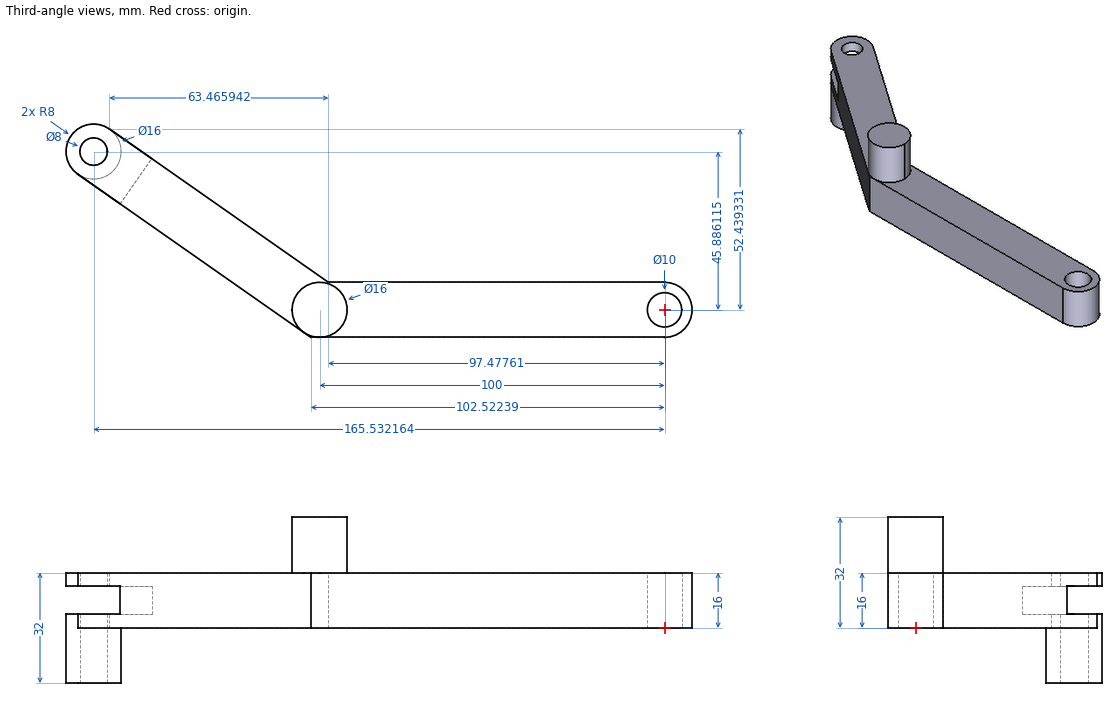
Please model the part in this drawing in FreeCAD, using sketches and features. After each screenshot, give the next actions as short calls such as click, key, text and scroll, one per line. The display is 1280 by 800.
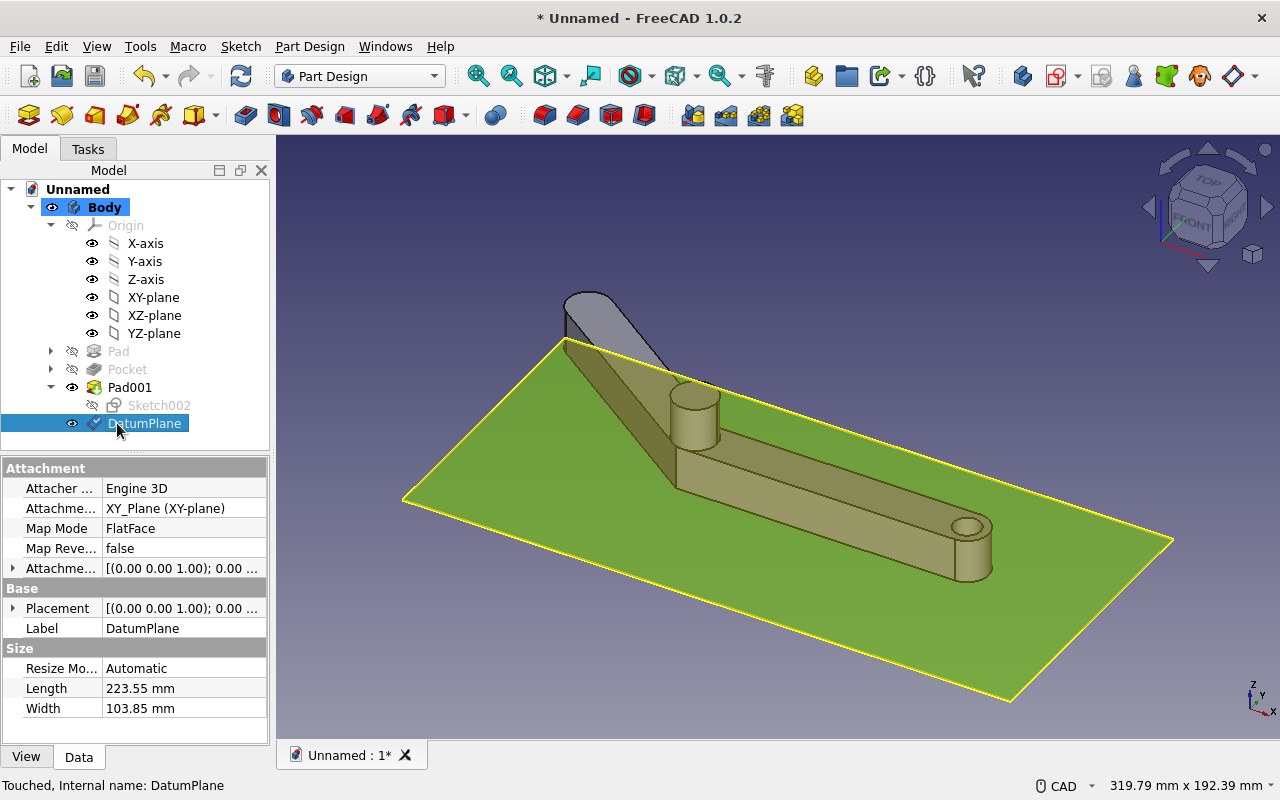
click(1056, 76)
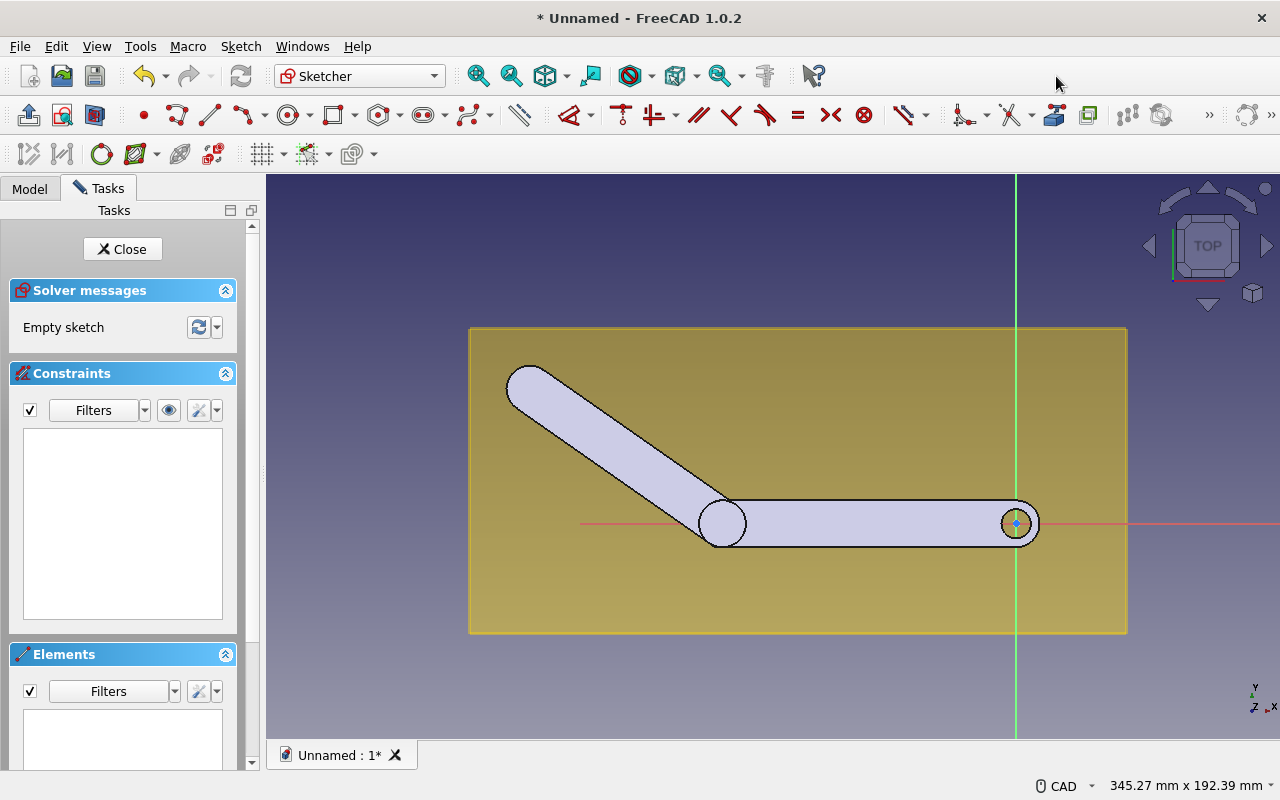
click(95, 116)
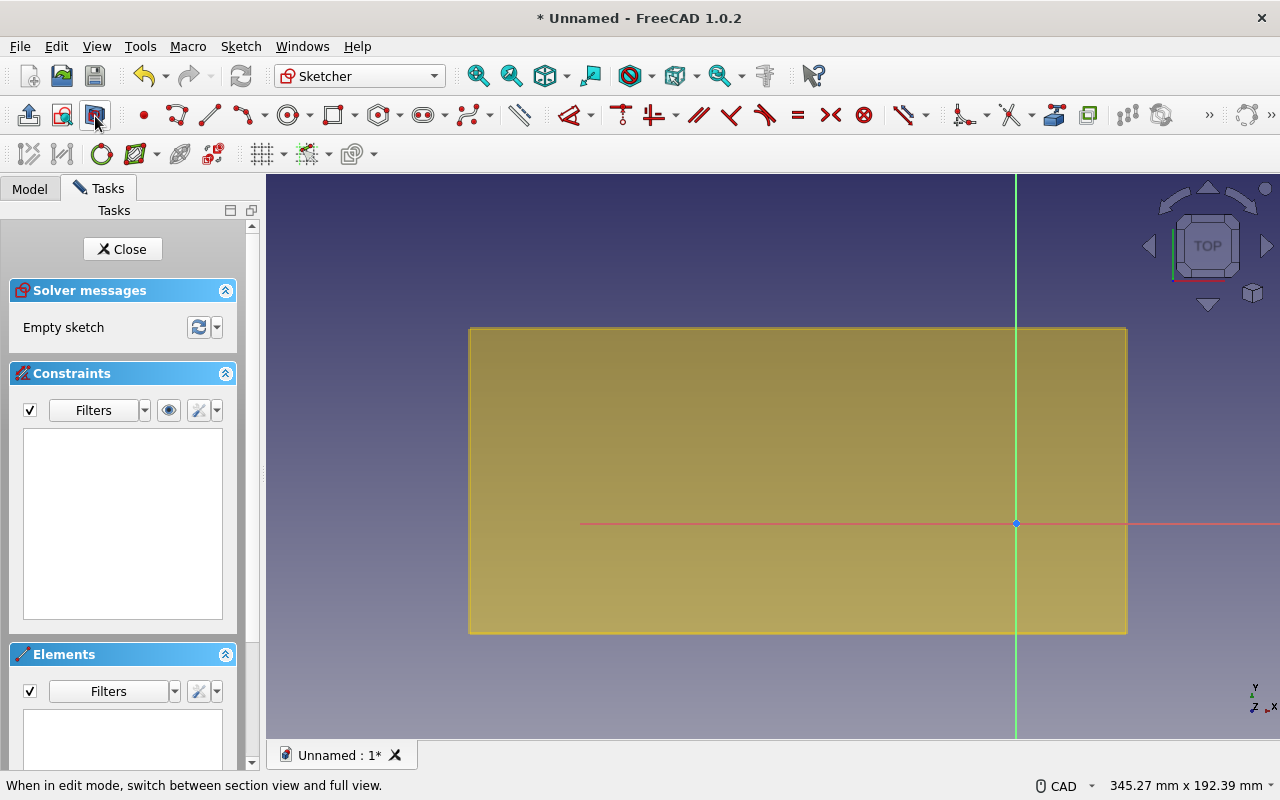
scroll(503, 378, up, 10)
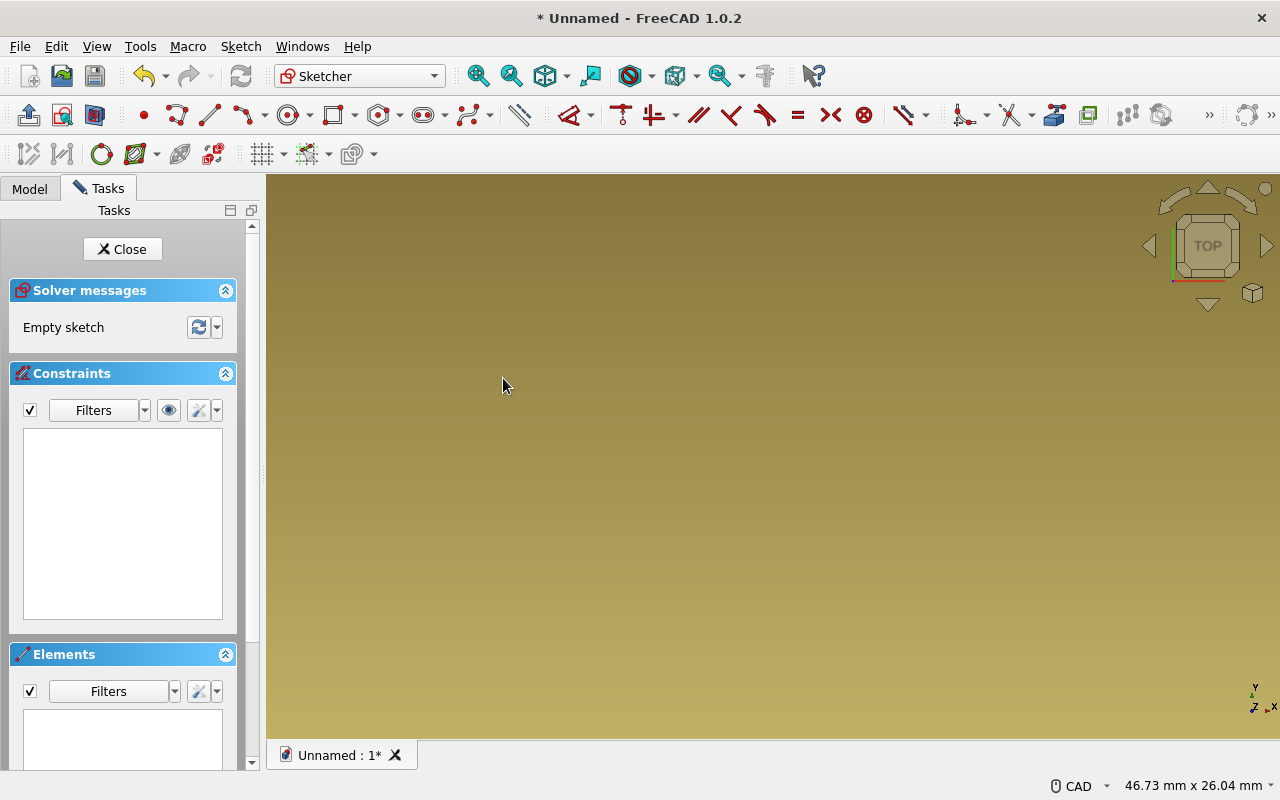
click(288, 116)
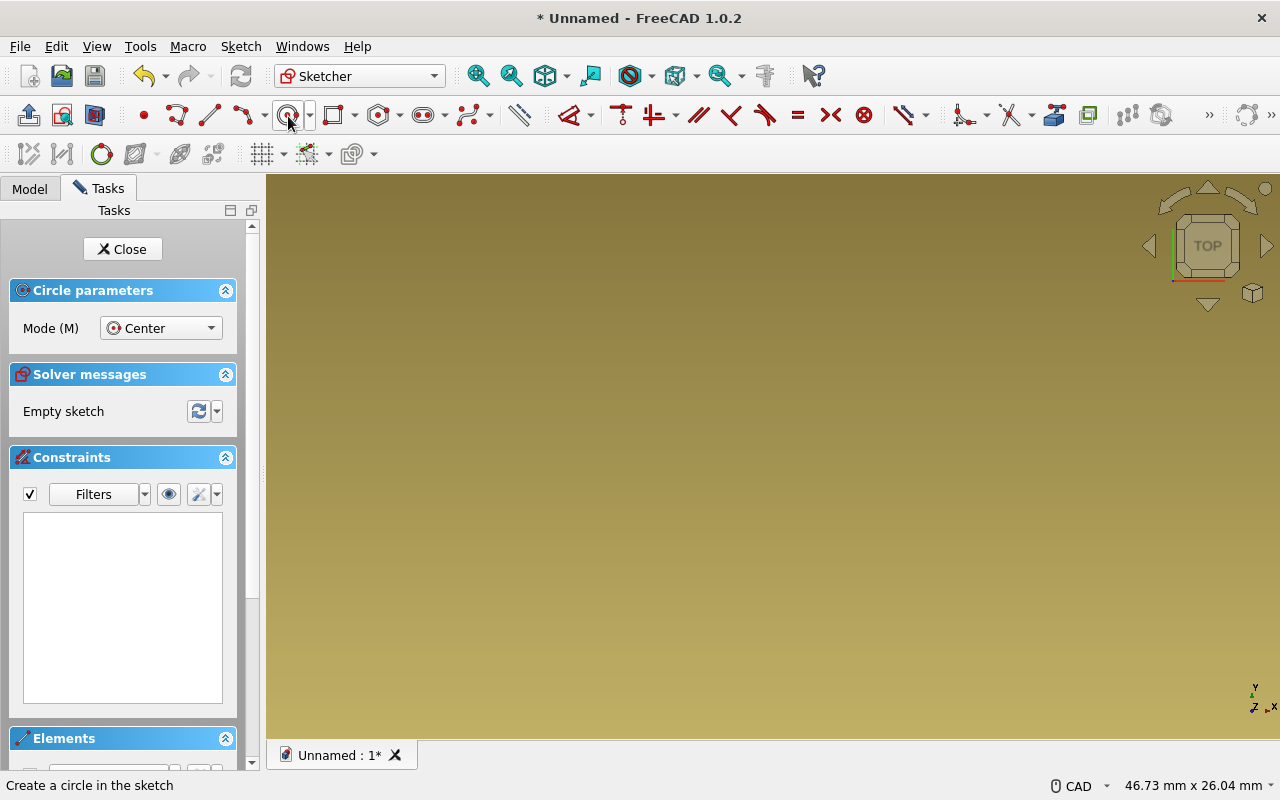
click(701, 457)
click(824, 335)
key(Escape)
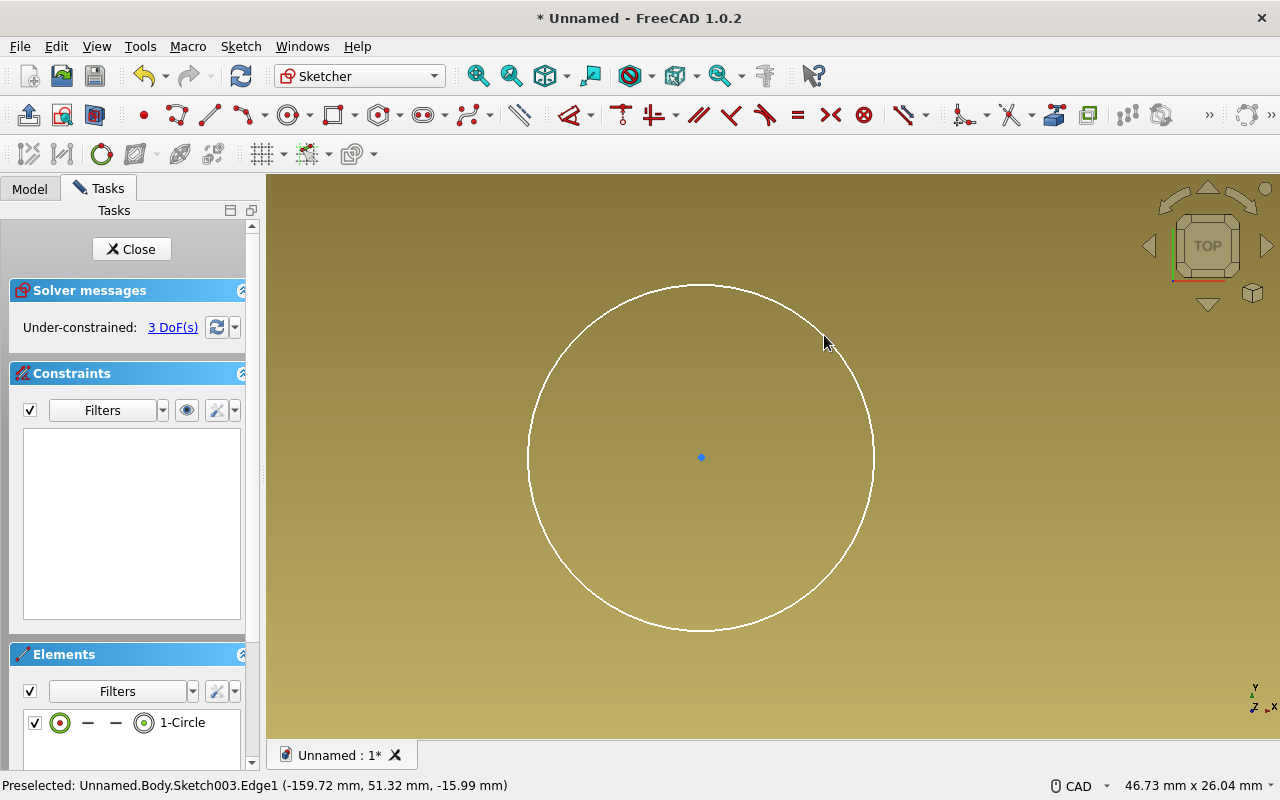
click(568, 116)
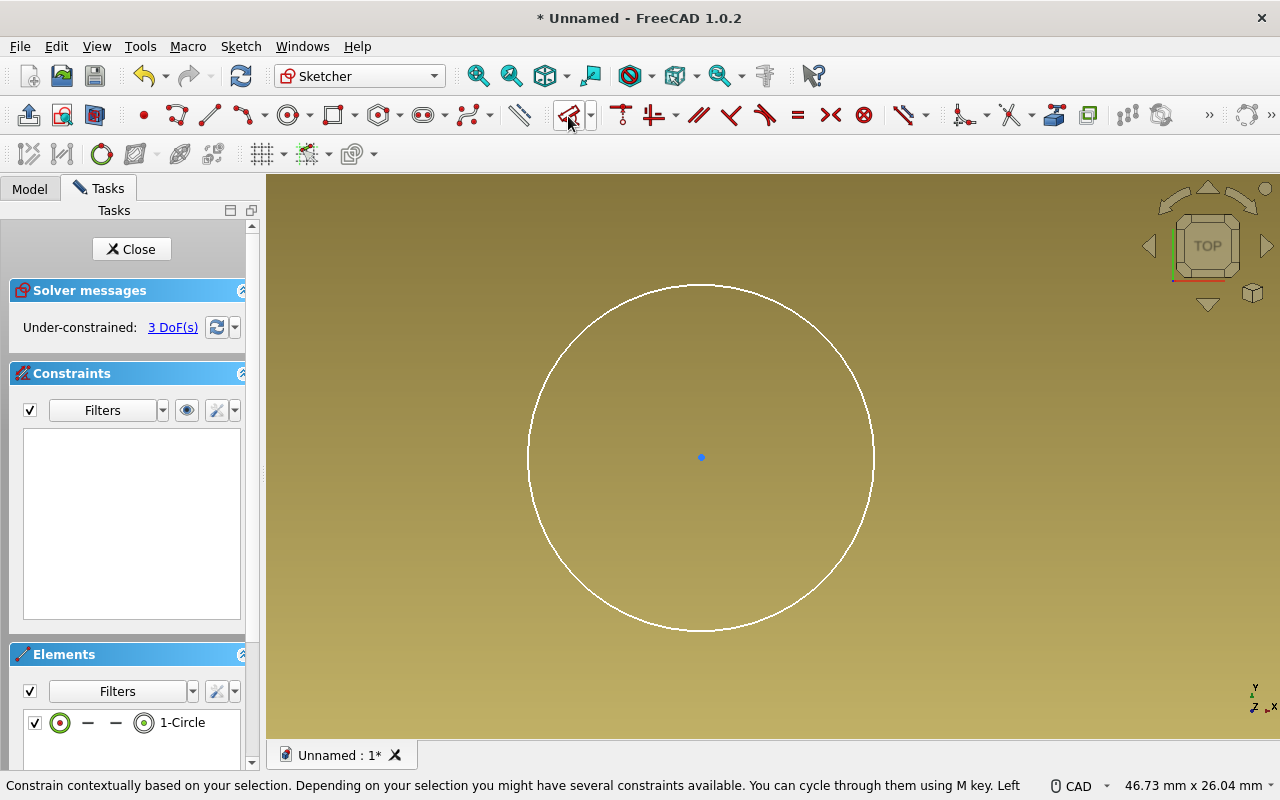
click(823, 335)
click(846, 312)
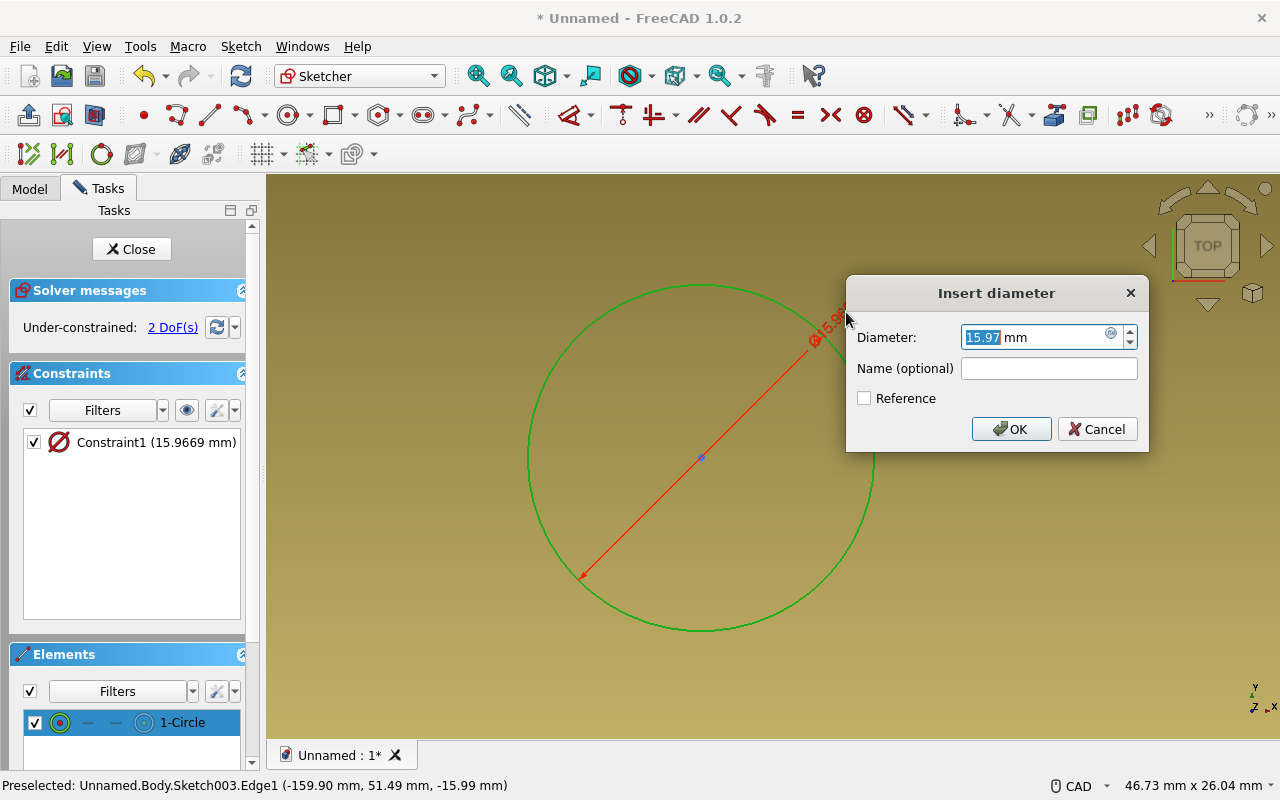
text(16)
key(Return)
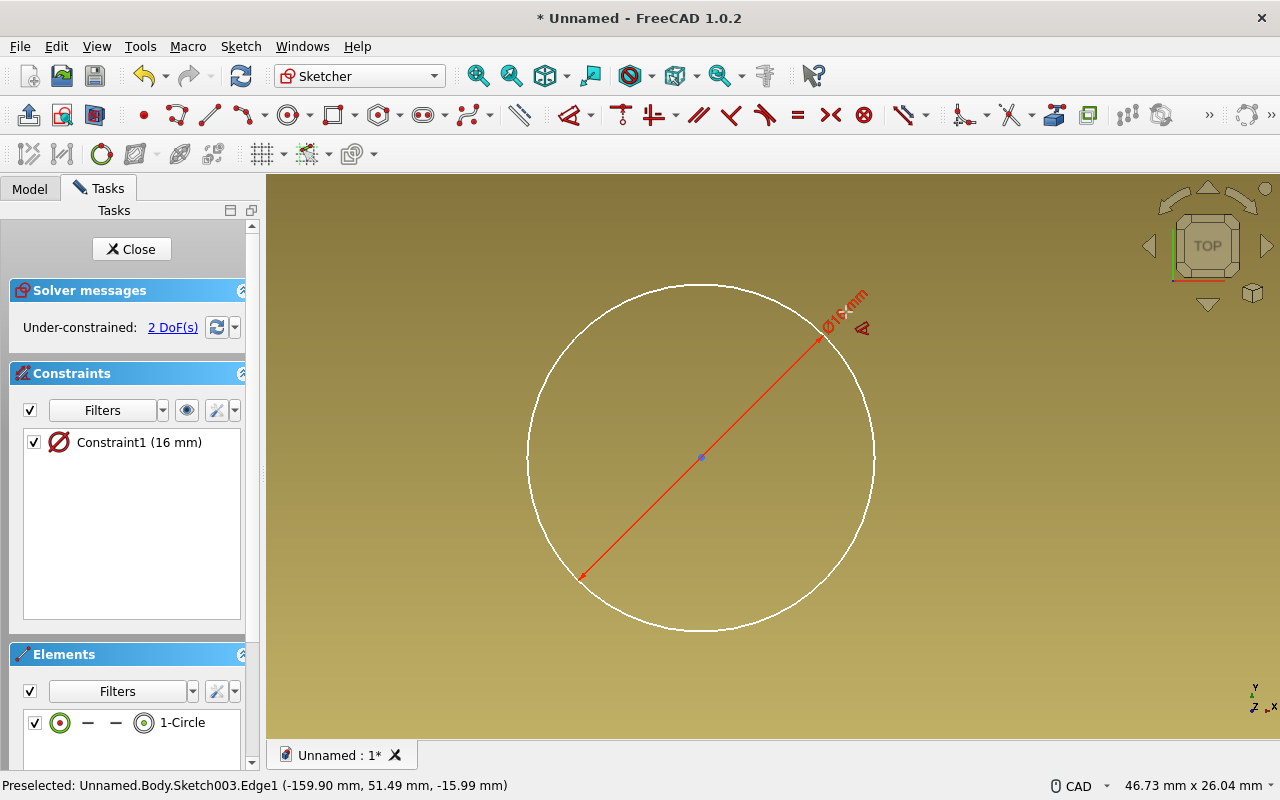
click(701, 458)
click(667, 584)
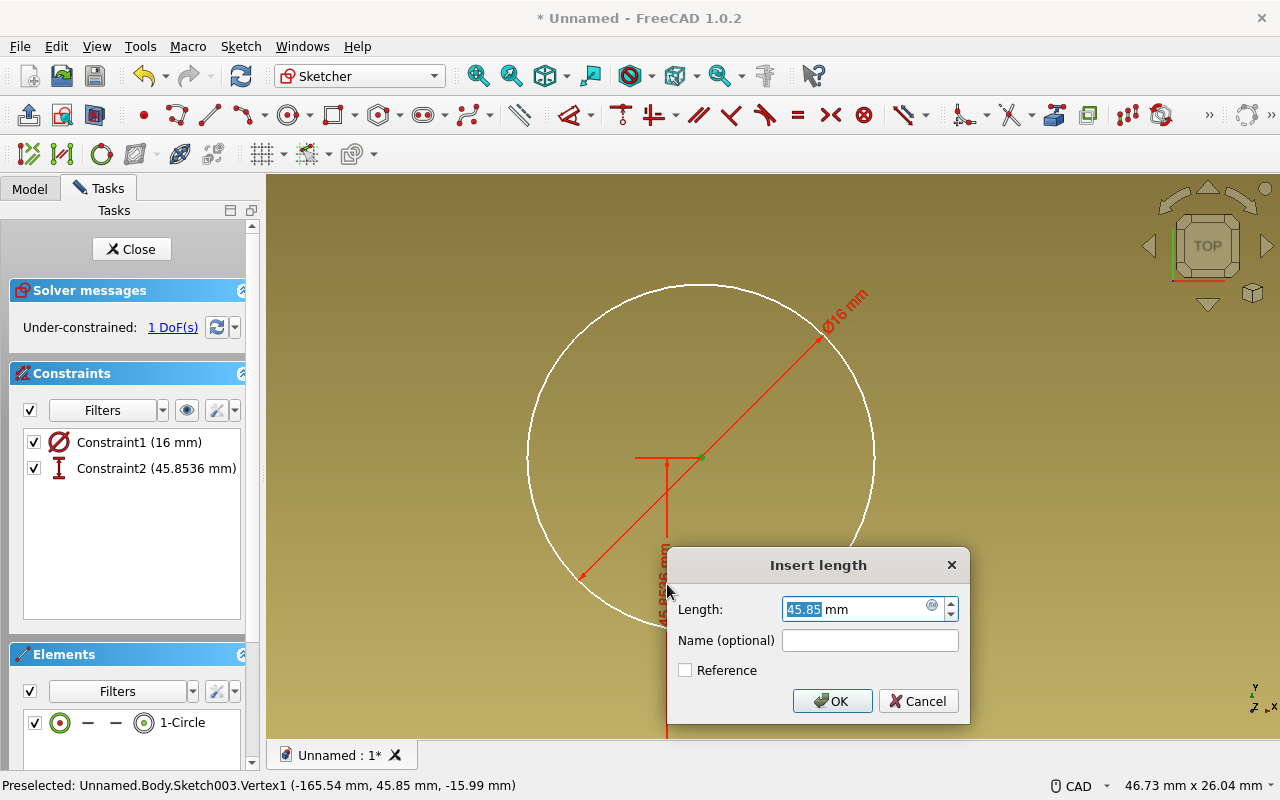
text(45.886115)
key(Return)